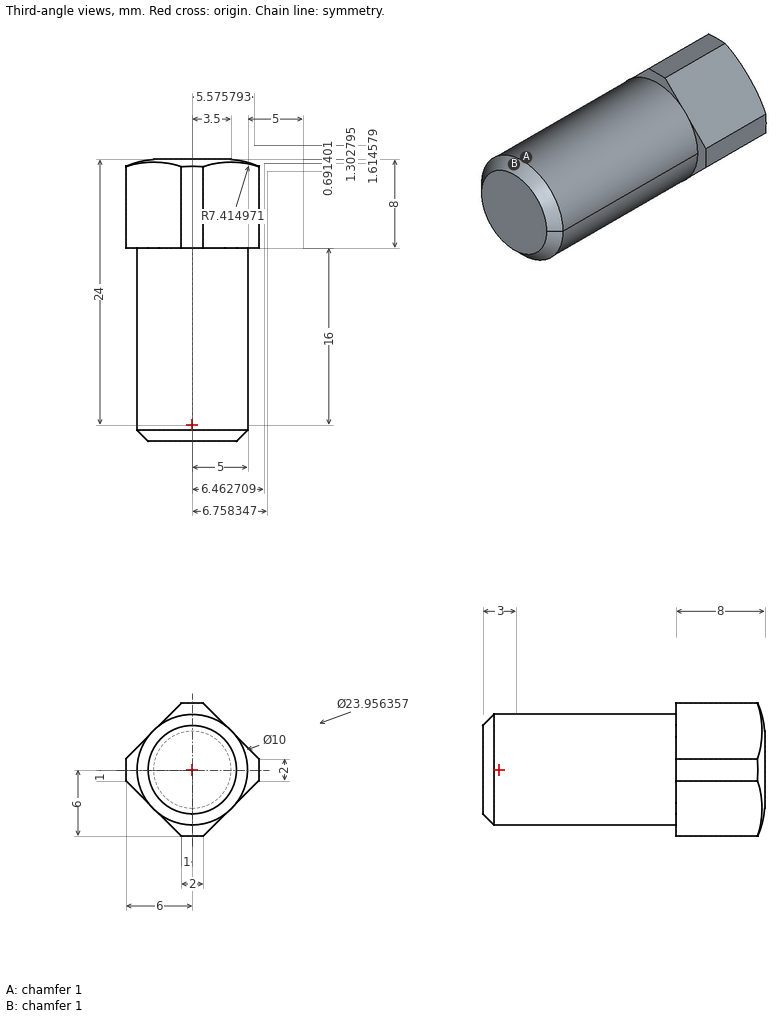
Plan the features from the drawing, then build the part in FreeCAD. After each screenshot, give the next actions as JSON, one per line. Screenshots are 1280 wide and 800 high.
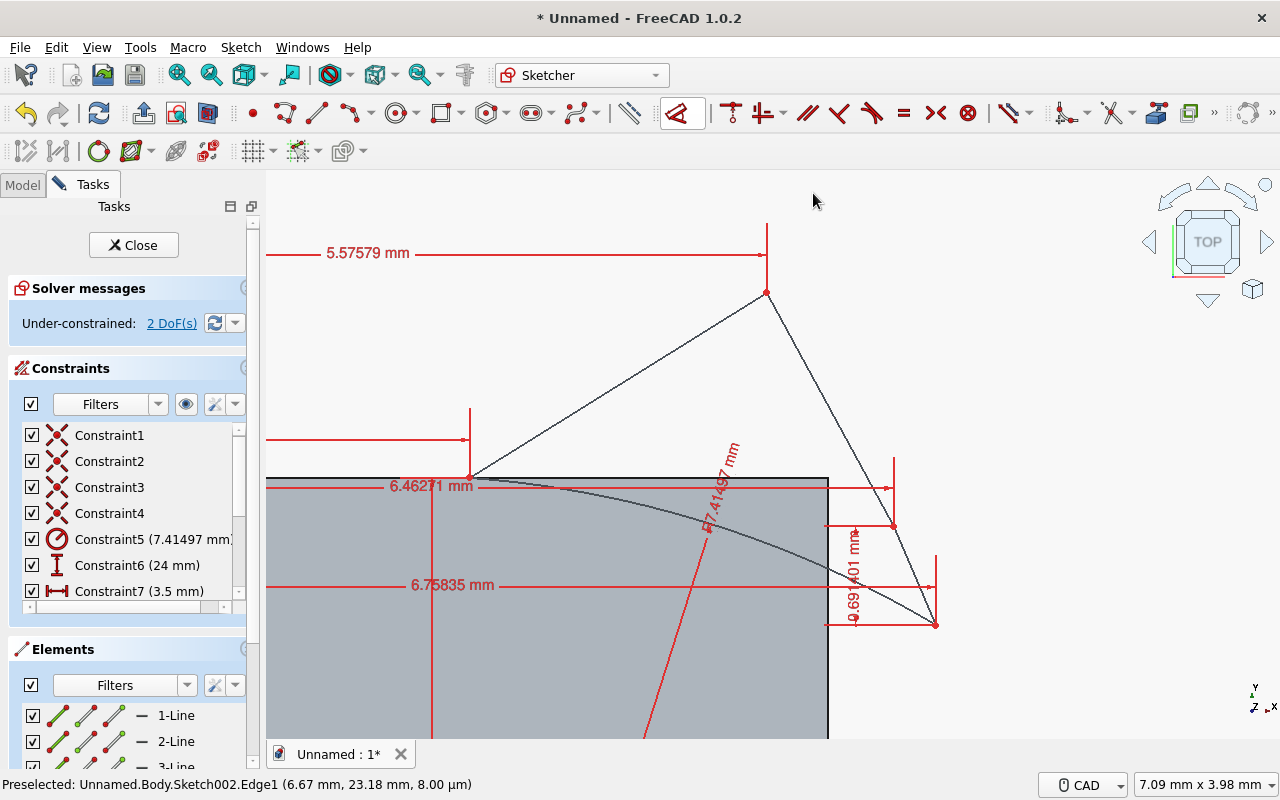
{"action": "left_click", "coordinate": [856, 456]}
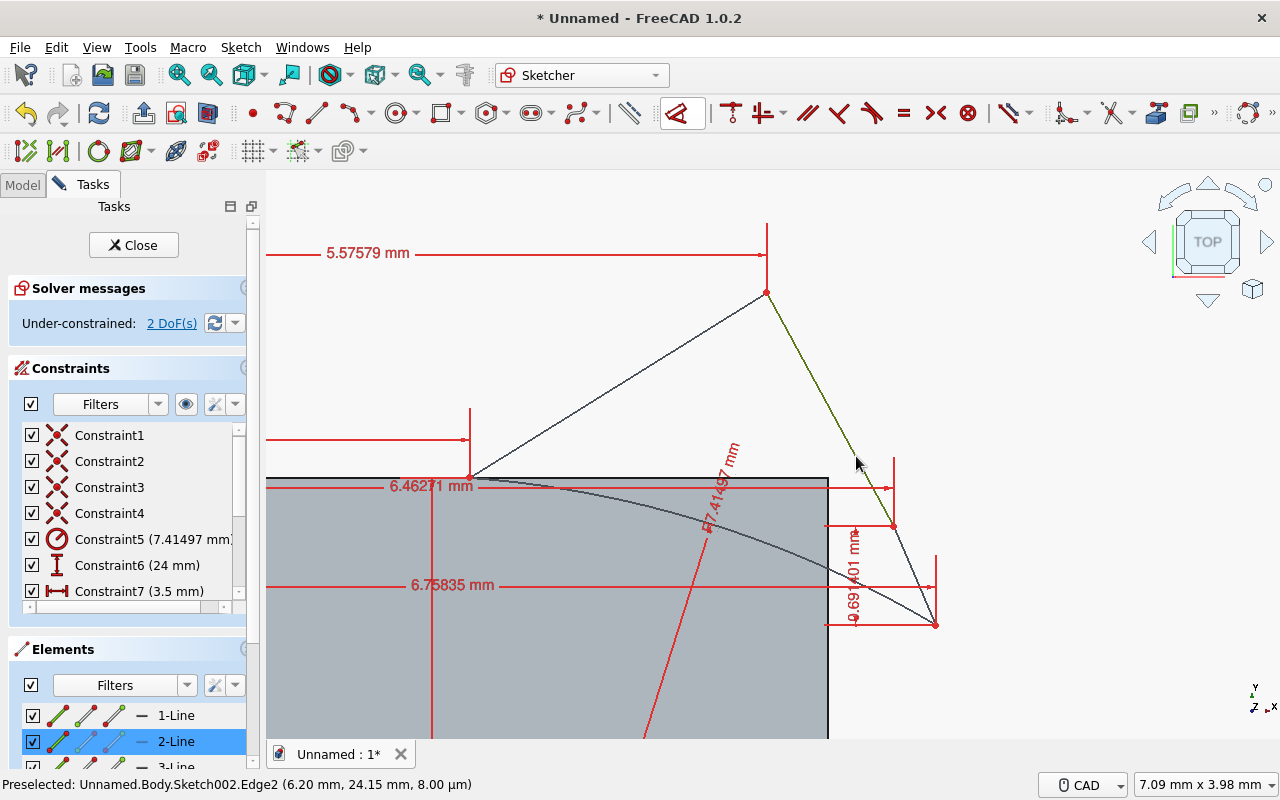
{"action": "left_click", "coordinate": [700, 114]}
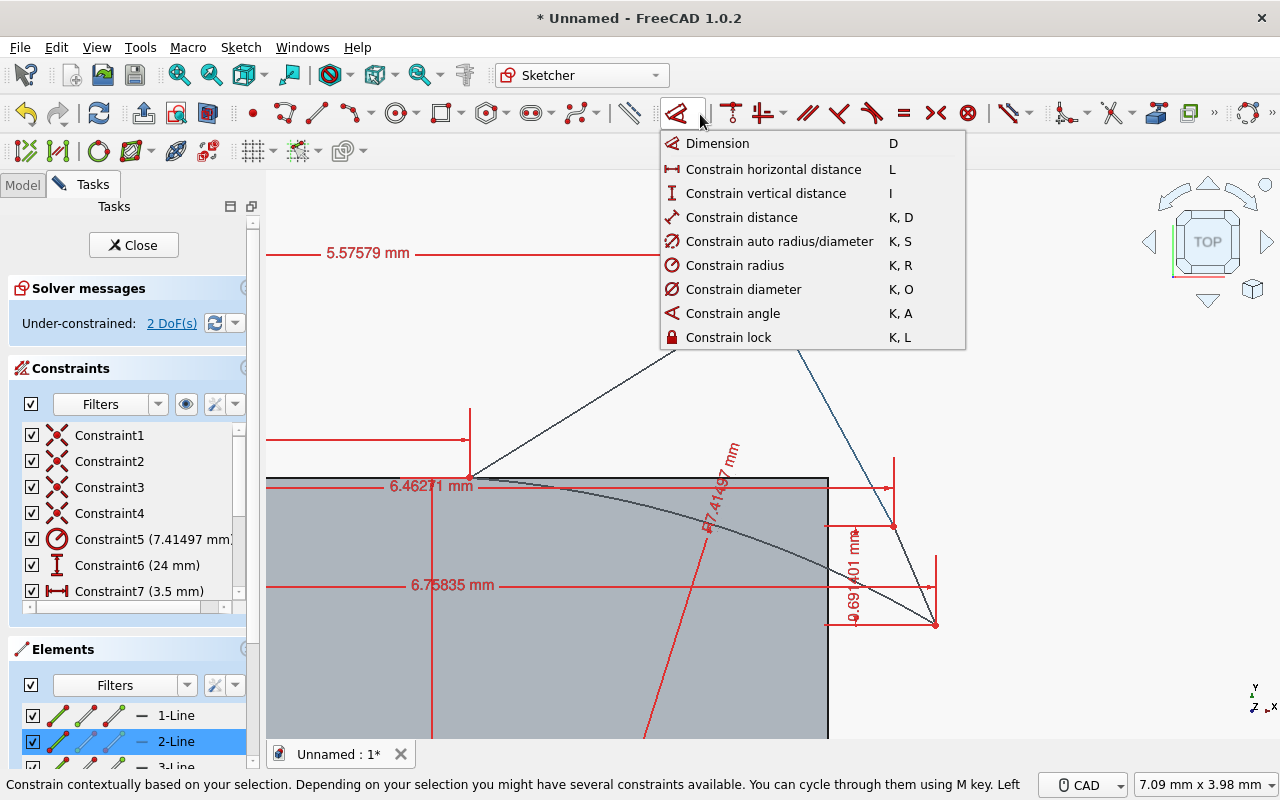
{"action": "left_click", "coordinate": [813, 193]}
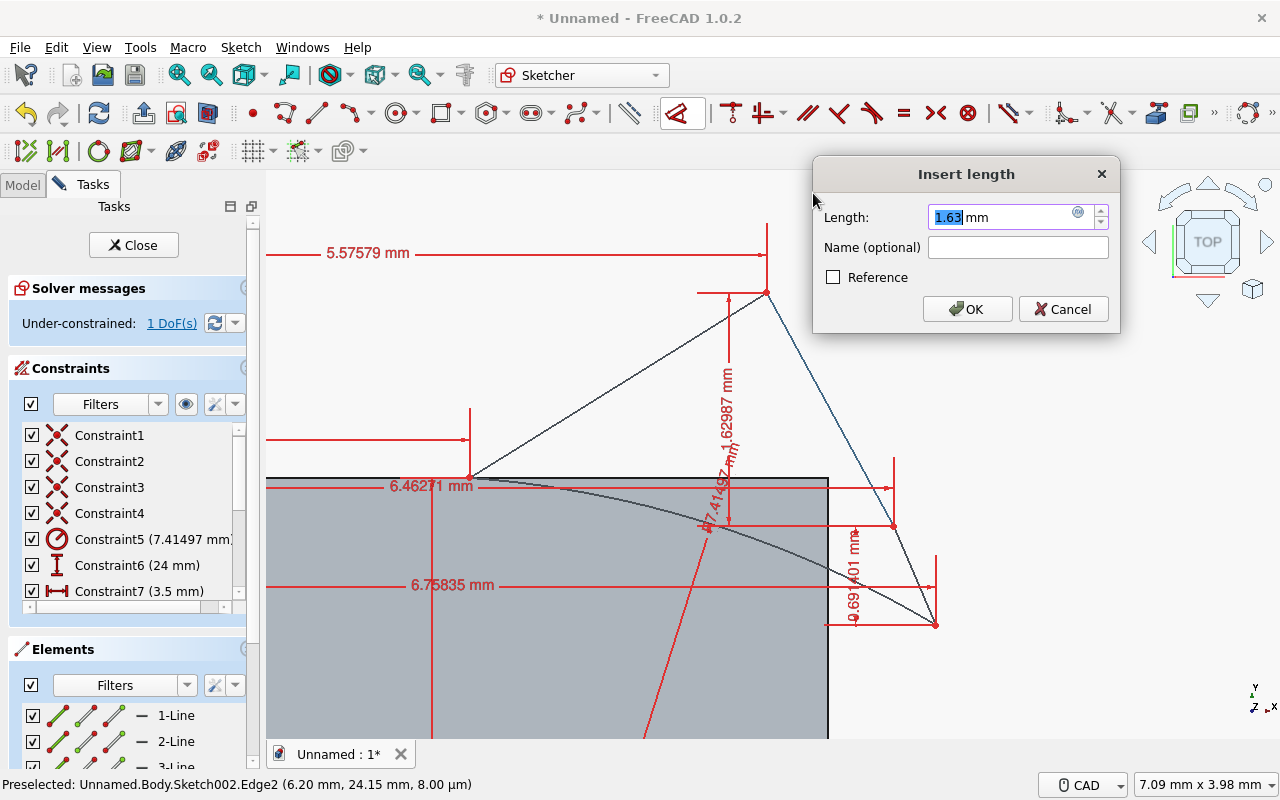
{"action": "type", "text": "1.614579"}
{"action": "key", "text": "Return"}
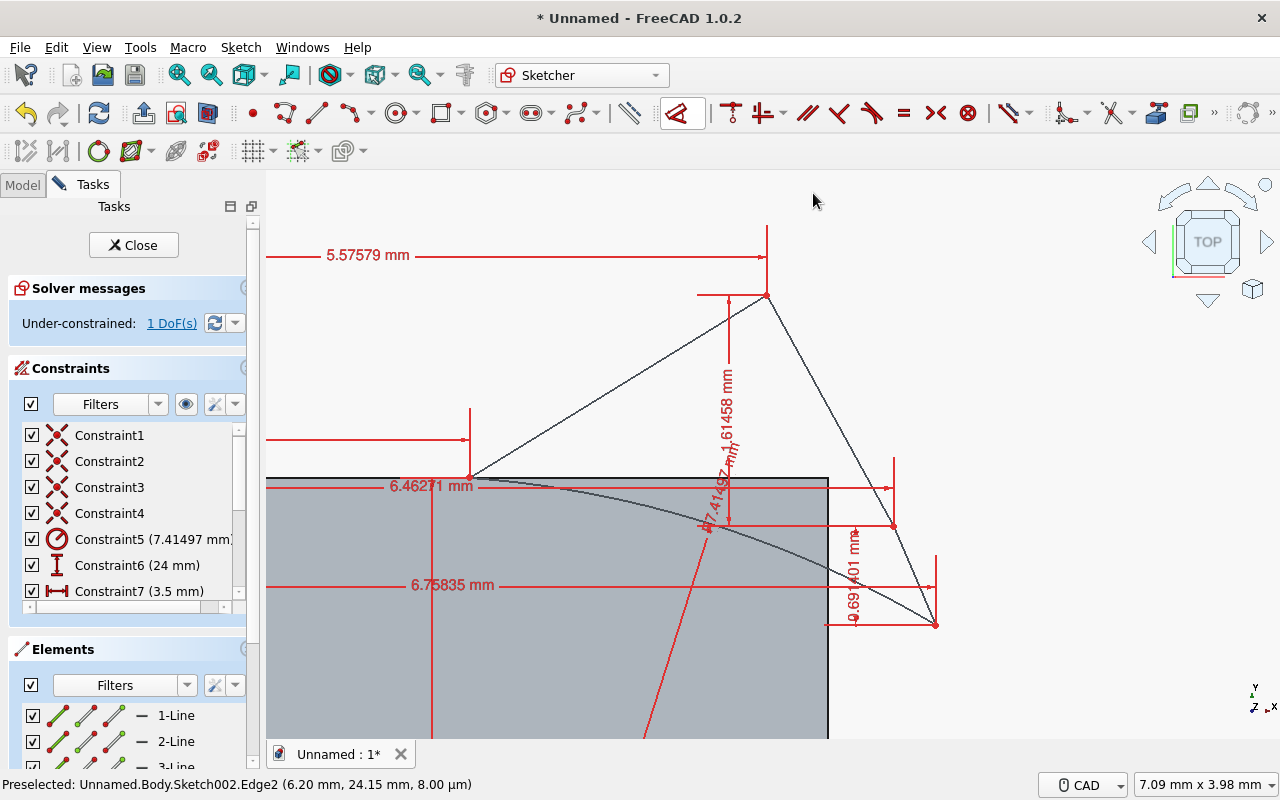
{"action": "left_click", "coordinate": [678, 350]}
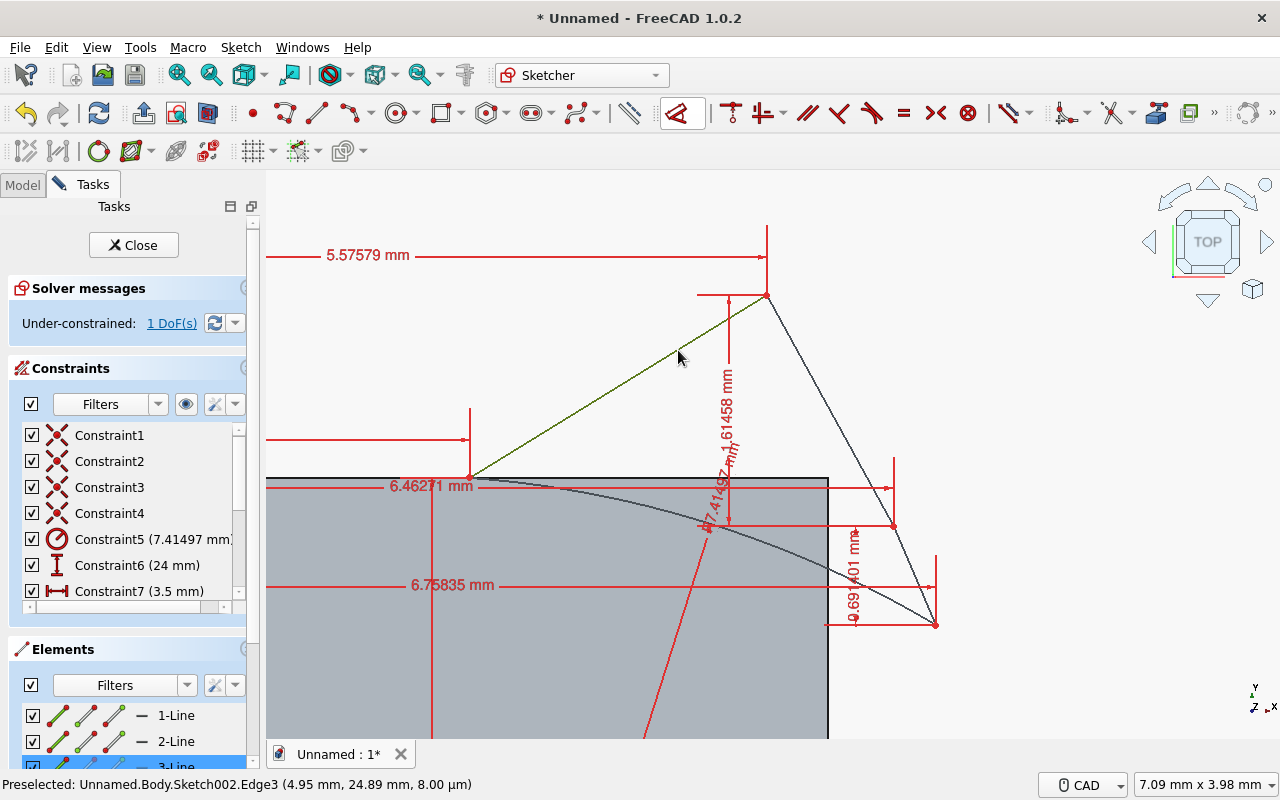
{"action": "left_click", "coordinate": [700, 114]}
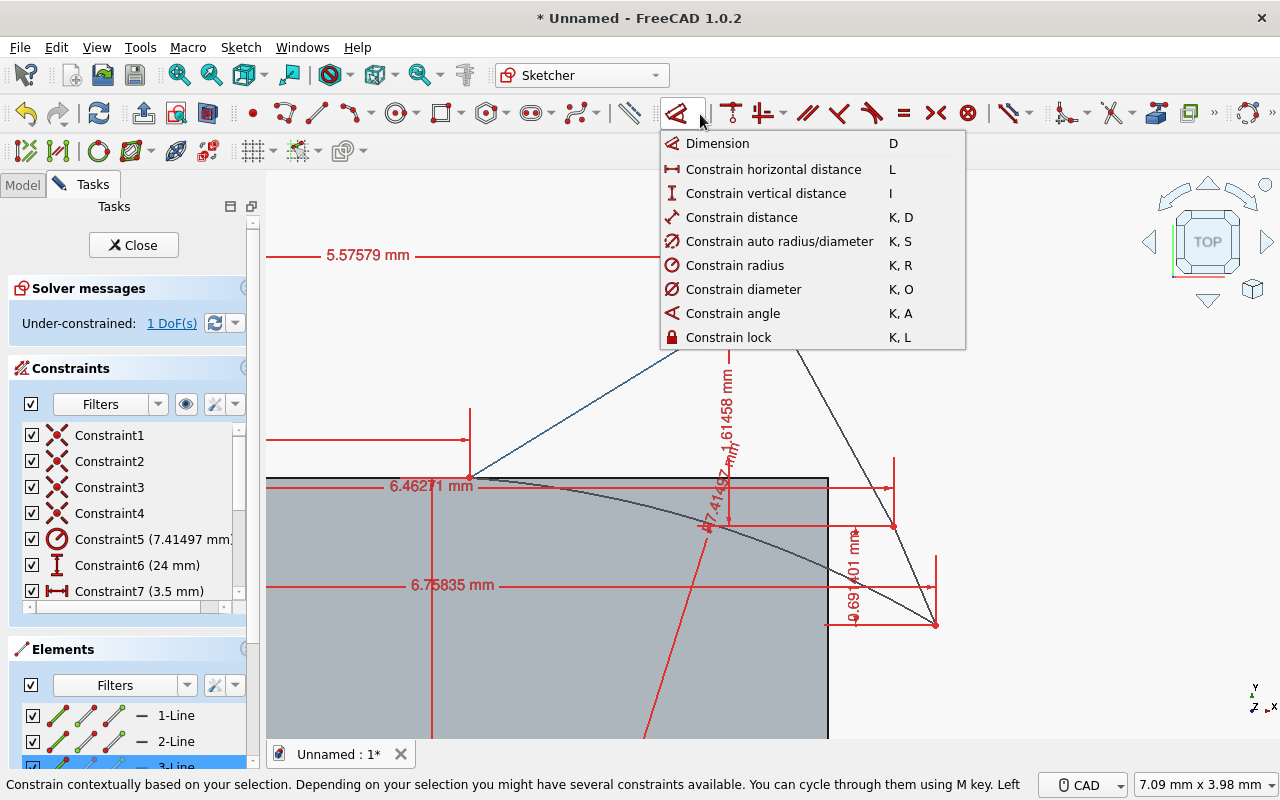
{"action": "left_click", "coordinate": [813, 193]}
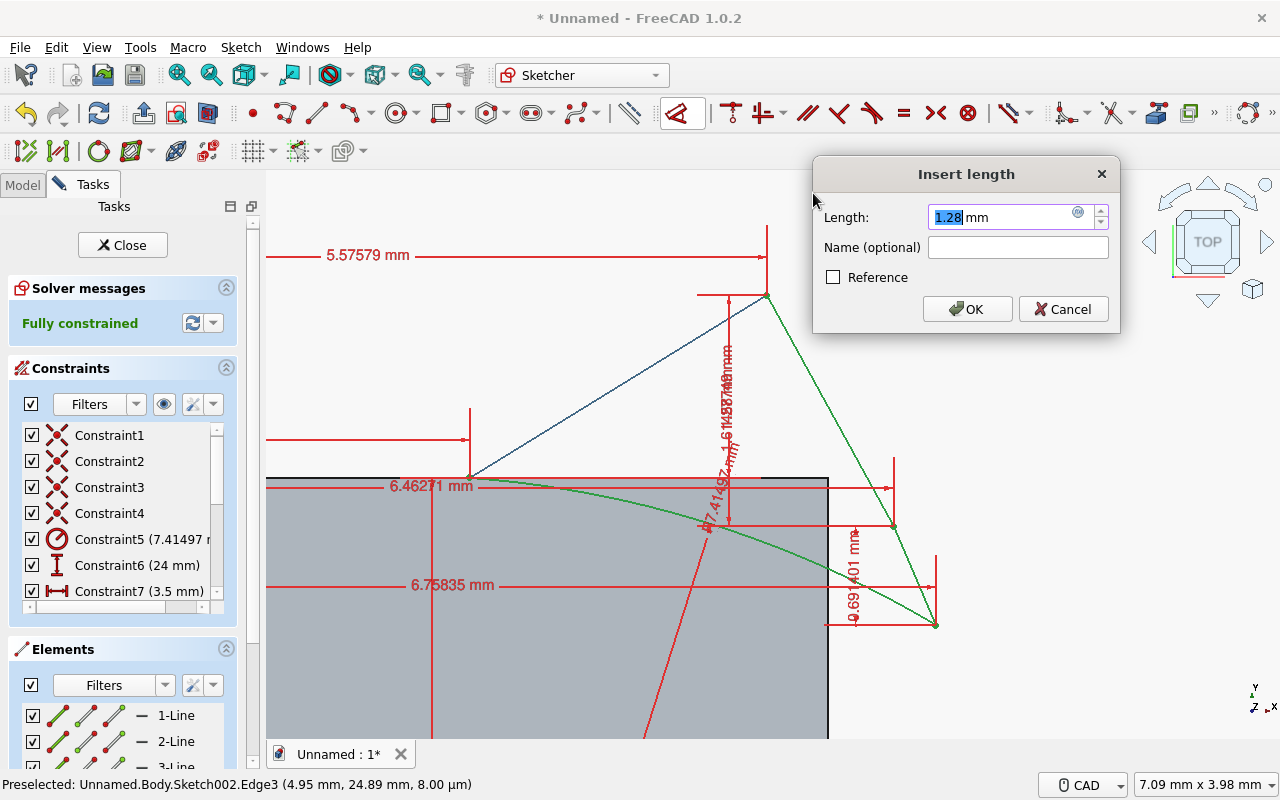
{"action": "type", "text": "1.302795"}
{"action": "key", "text": "Return"}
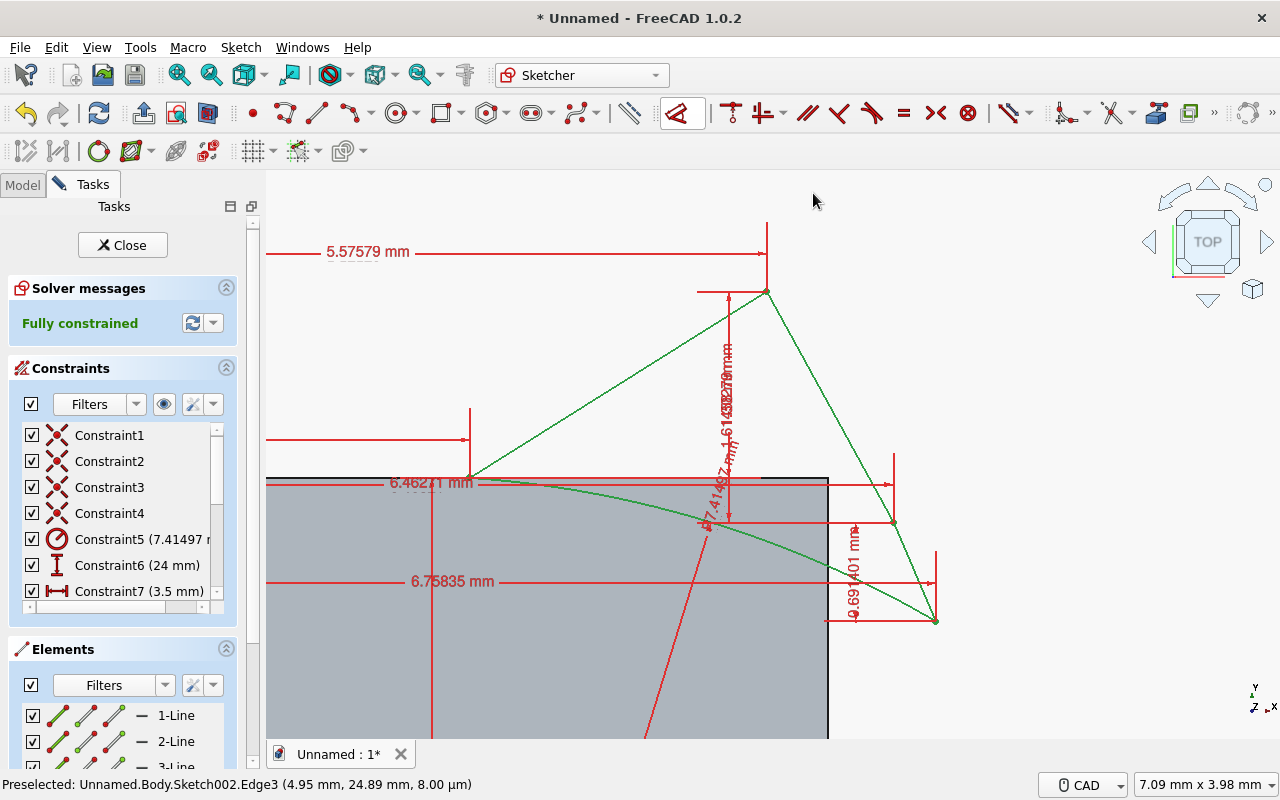
{"action": "left_click", "coordinate": [123, 245]}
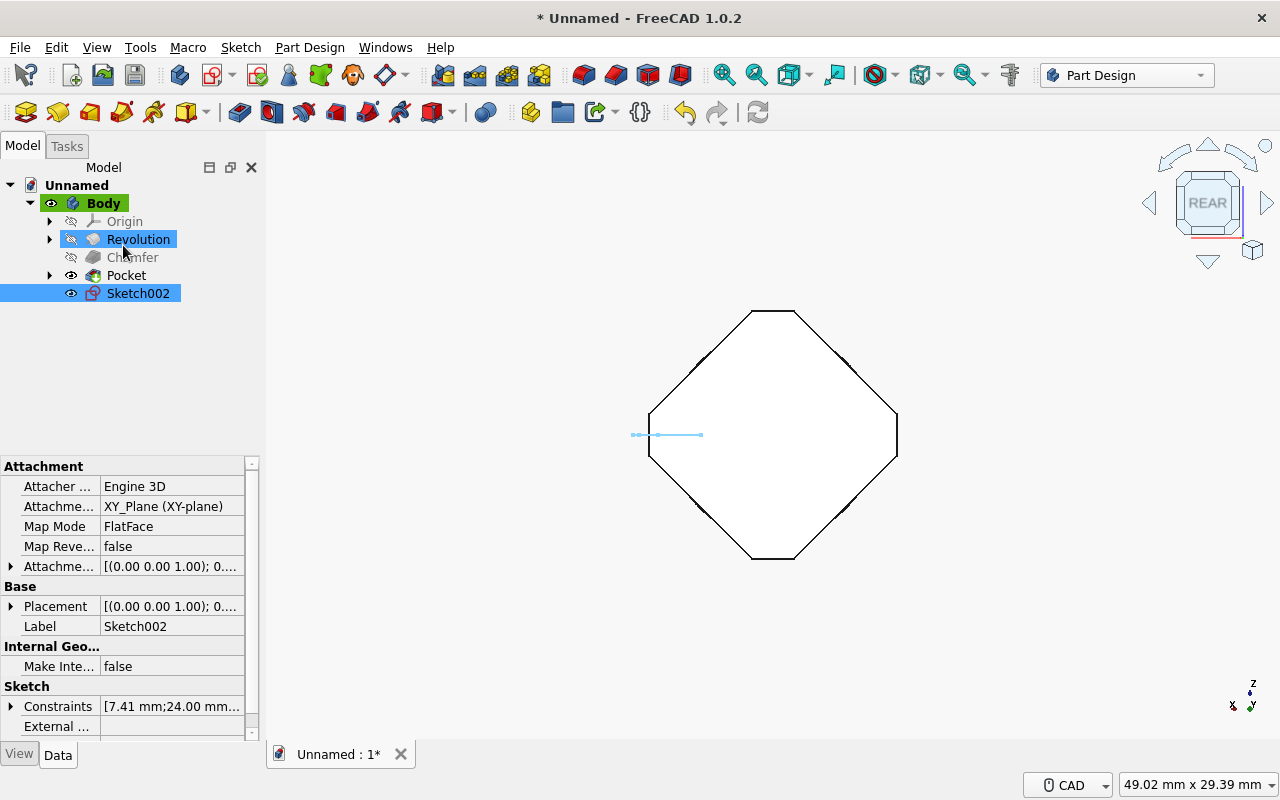
{"action": "left_click", "coordinate": [304, 112]}